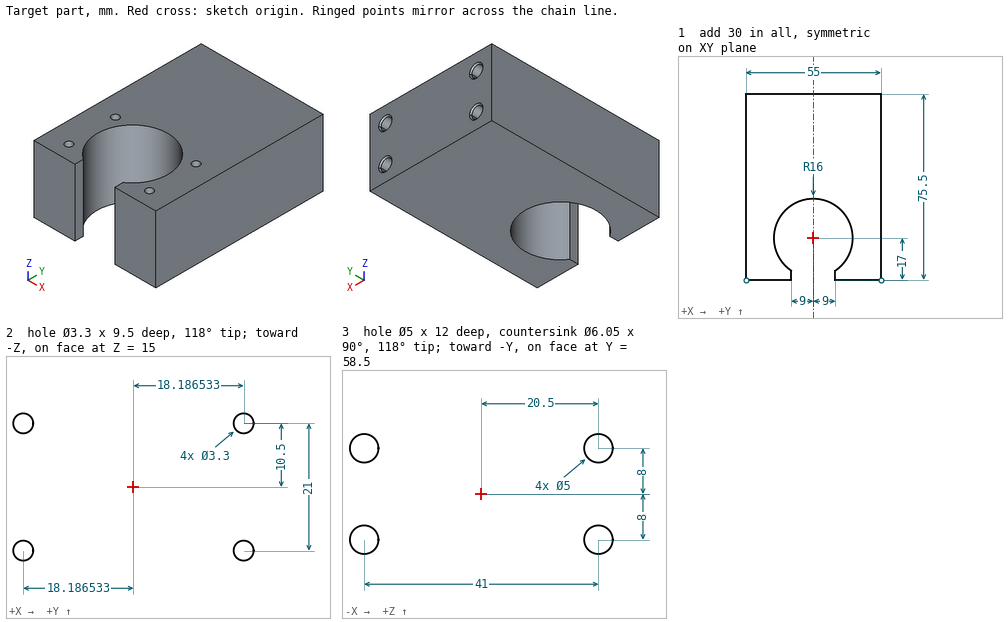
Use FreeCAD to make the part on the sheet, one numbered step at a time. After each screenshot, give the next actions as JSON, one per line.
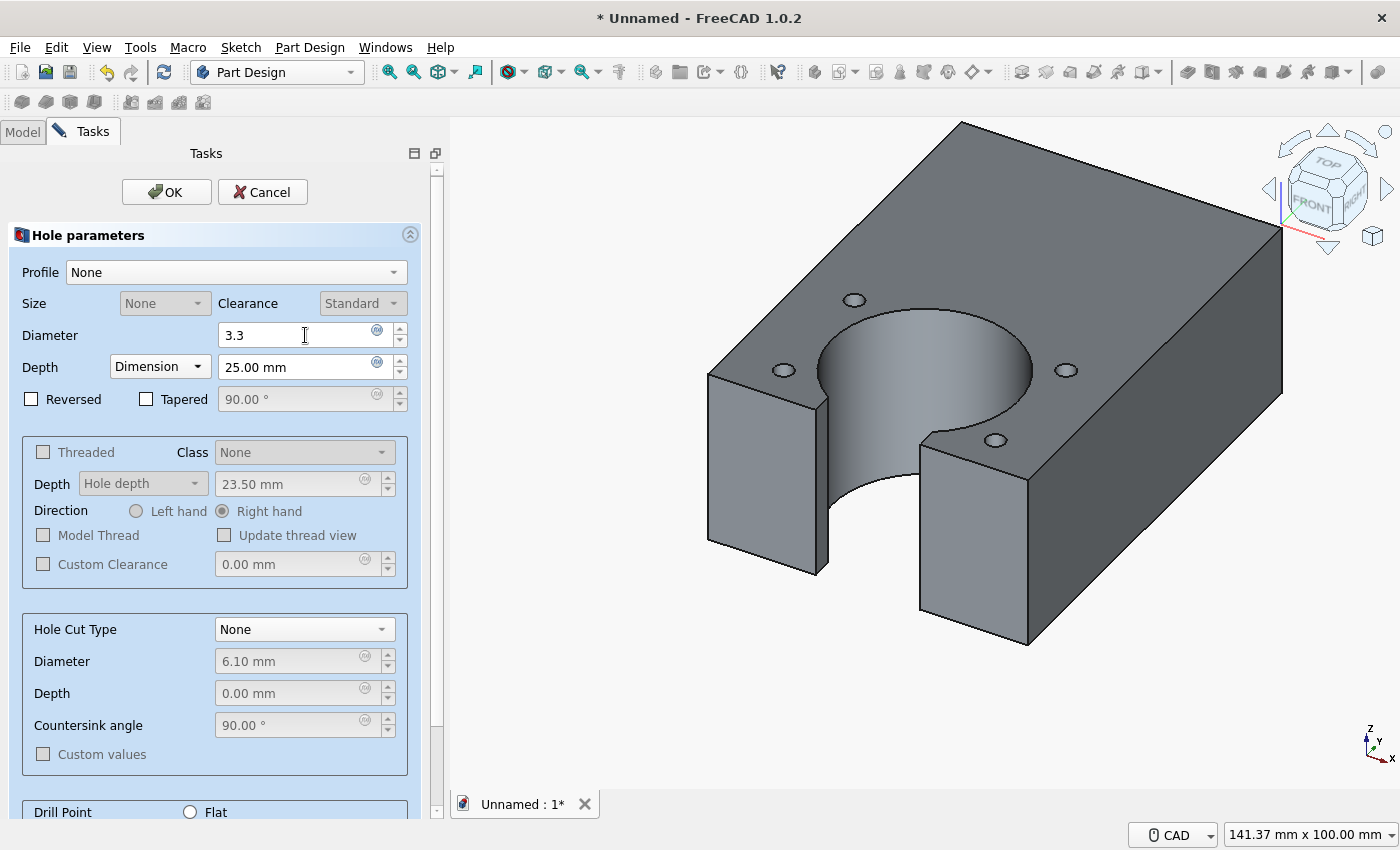
{"action": "triple_click", "coordinate": [305, 367]}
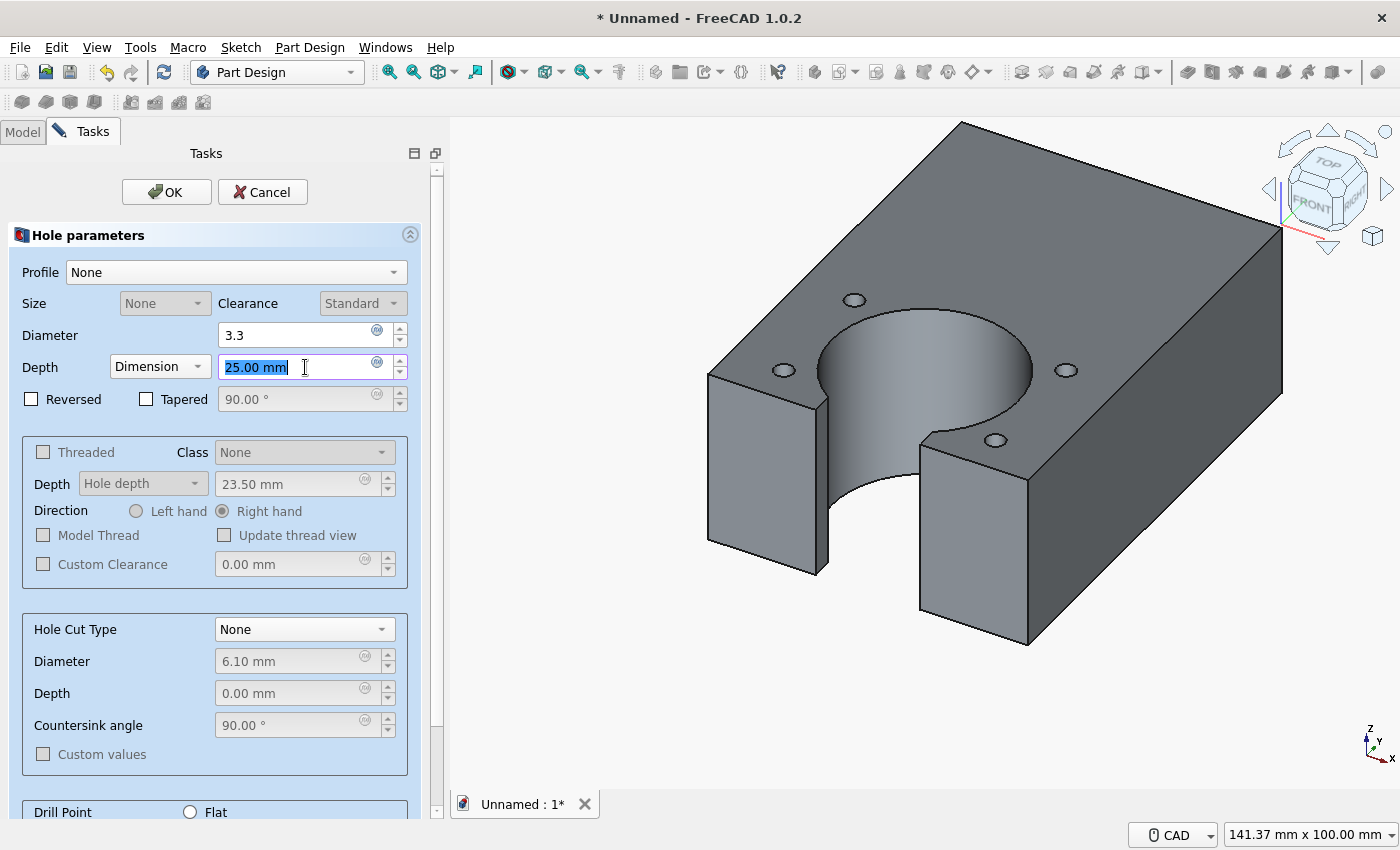
{"action": "type", "text": "9.5"}
{"action": "key", "text": "Tab"}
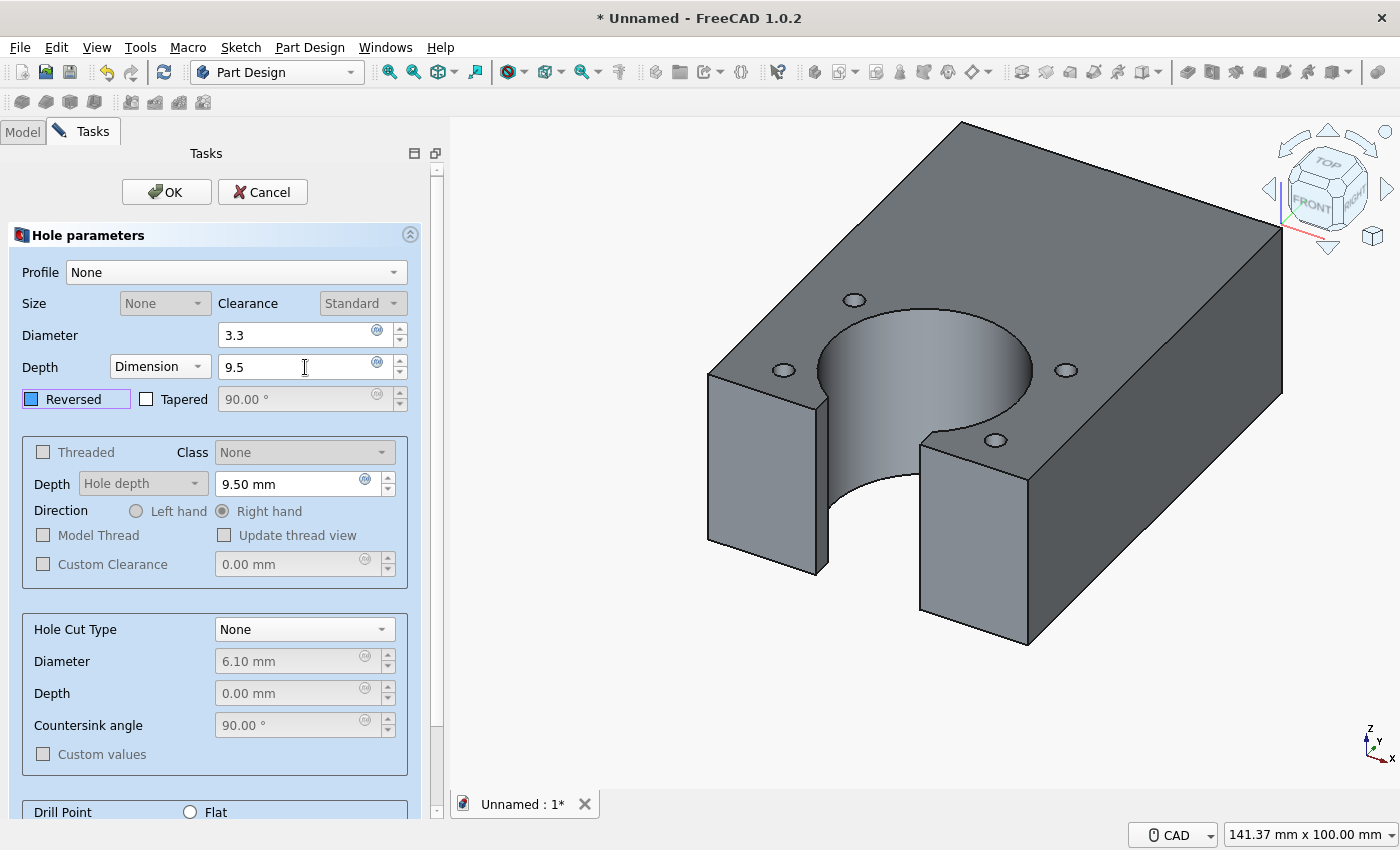
{"action": "left_click", "coordinate": [167, 192]}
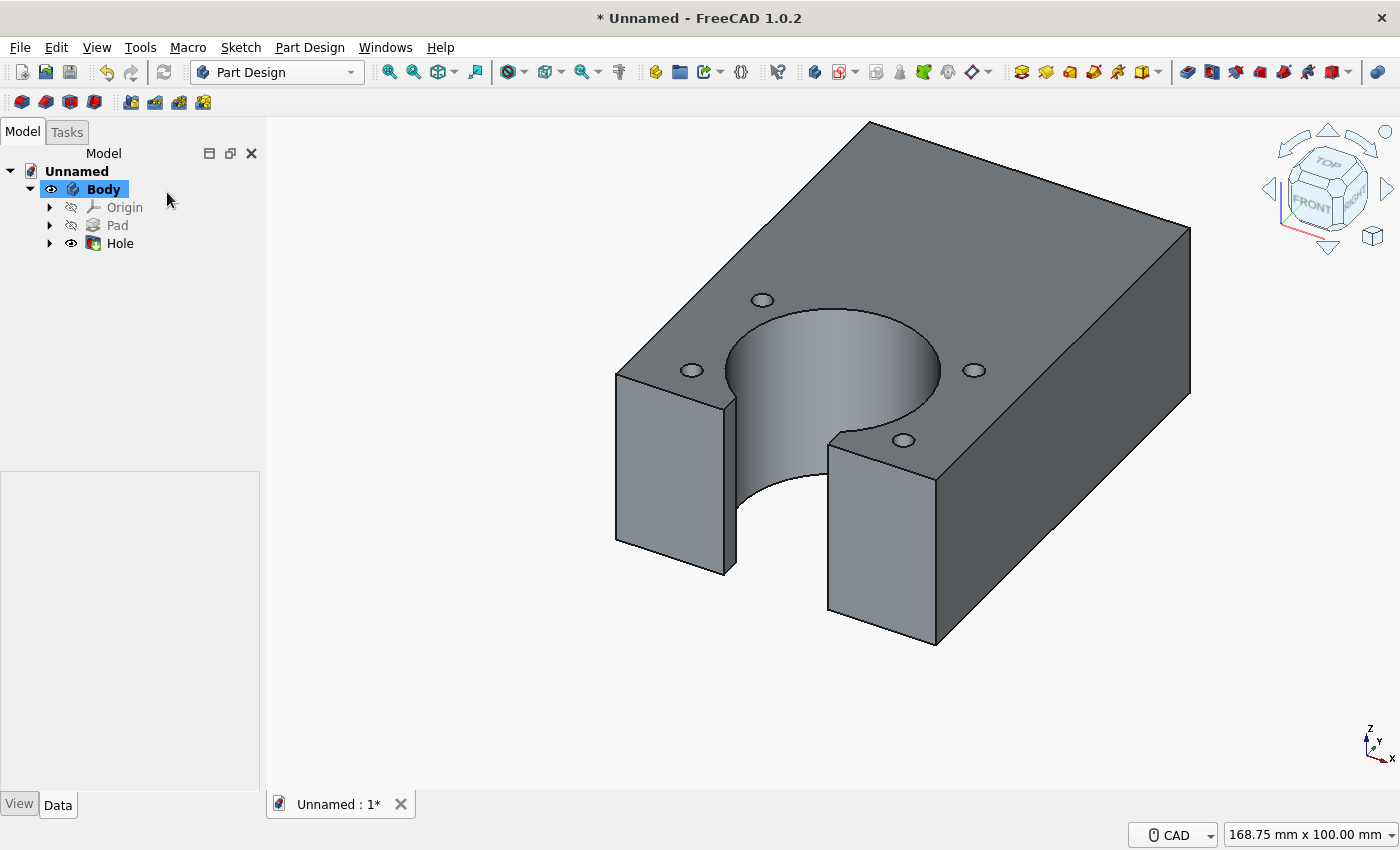
{"action": "key", "text": "4"}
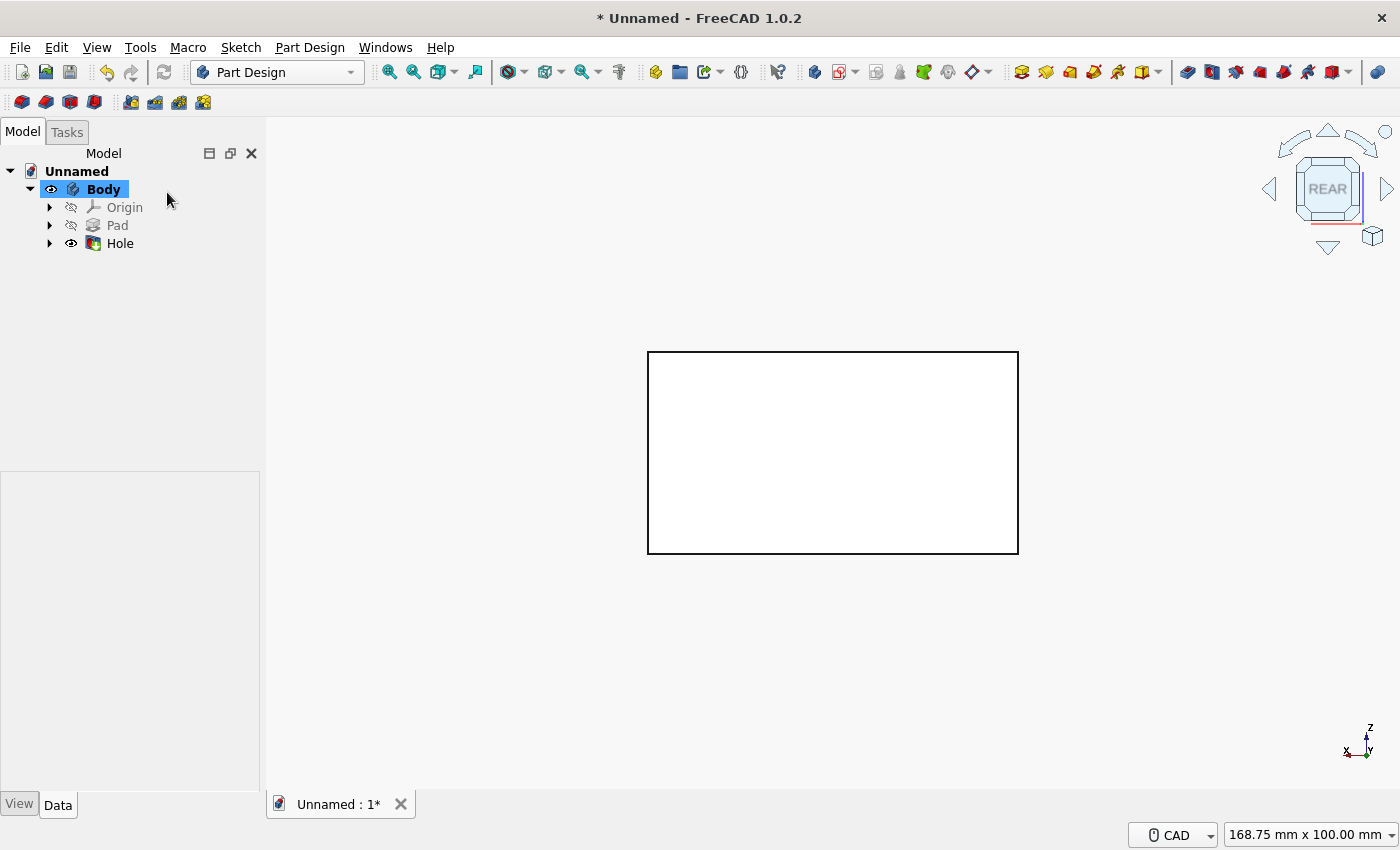
{"action": "left_click", "coordinate": [390, 72]}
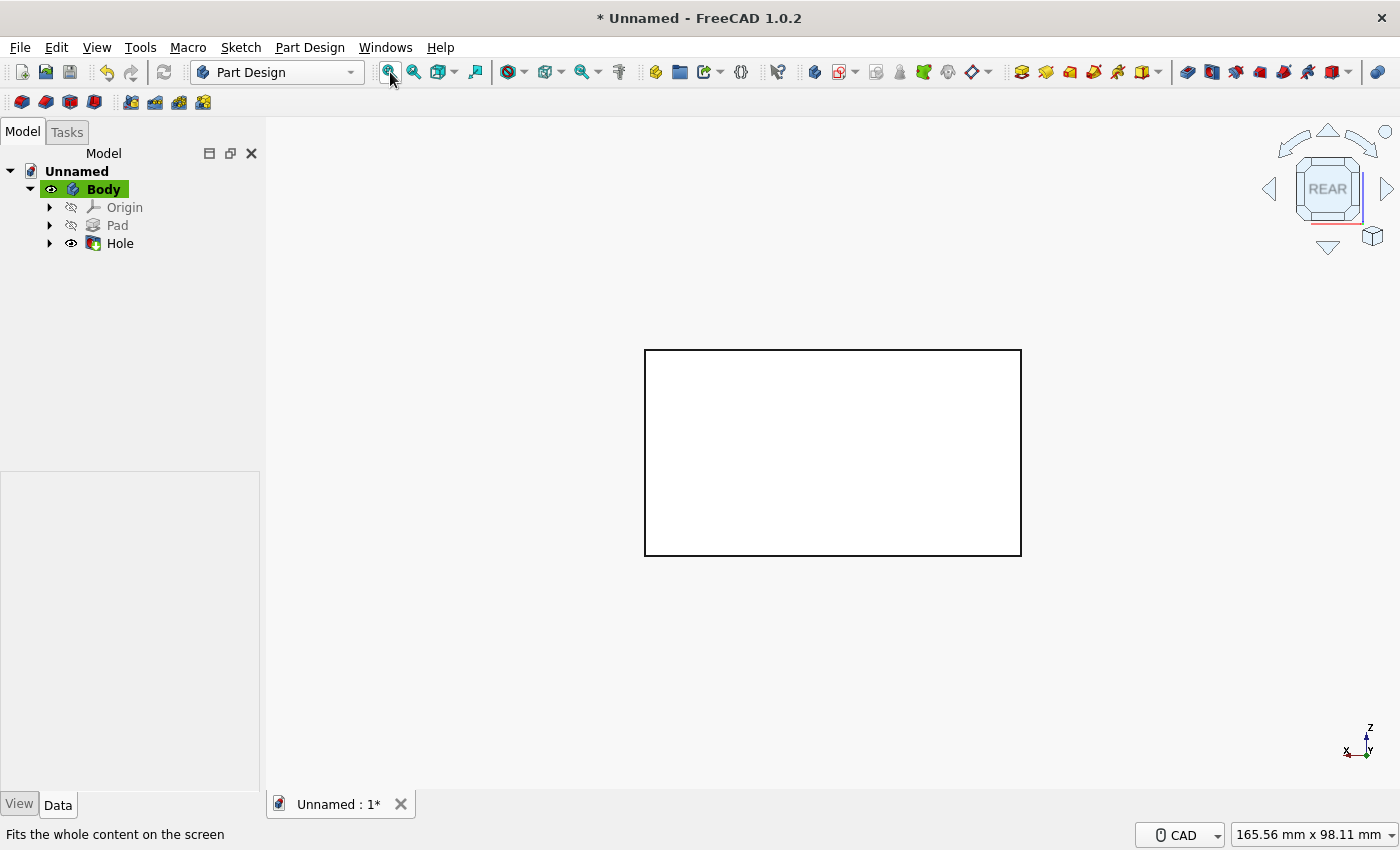
{"action": "left_click", "coordinate": [779, 452]}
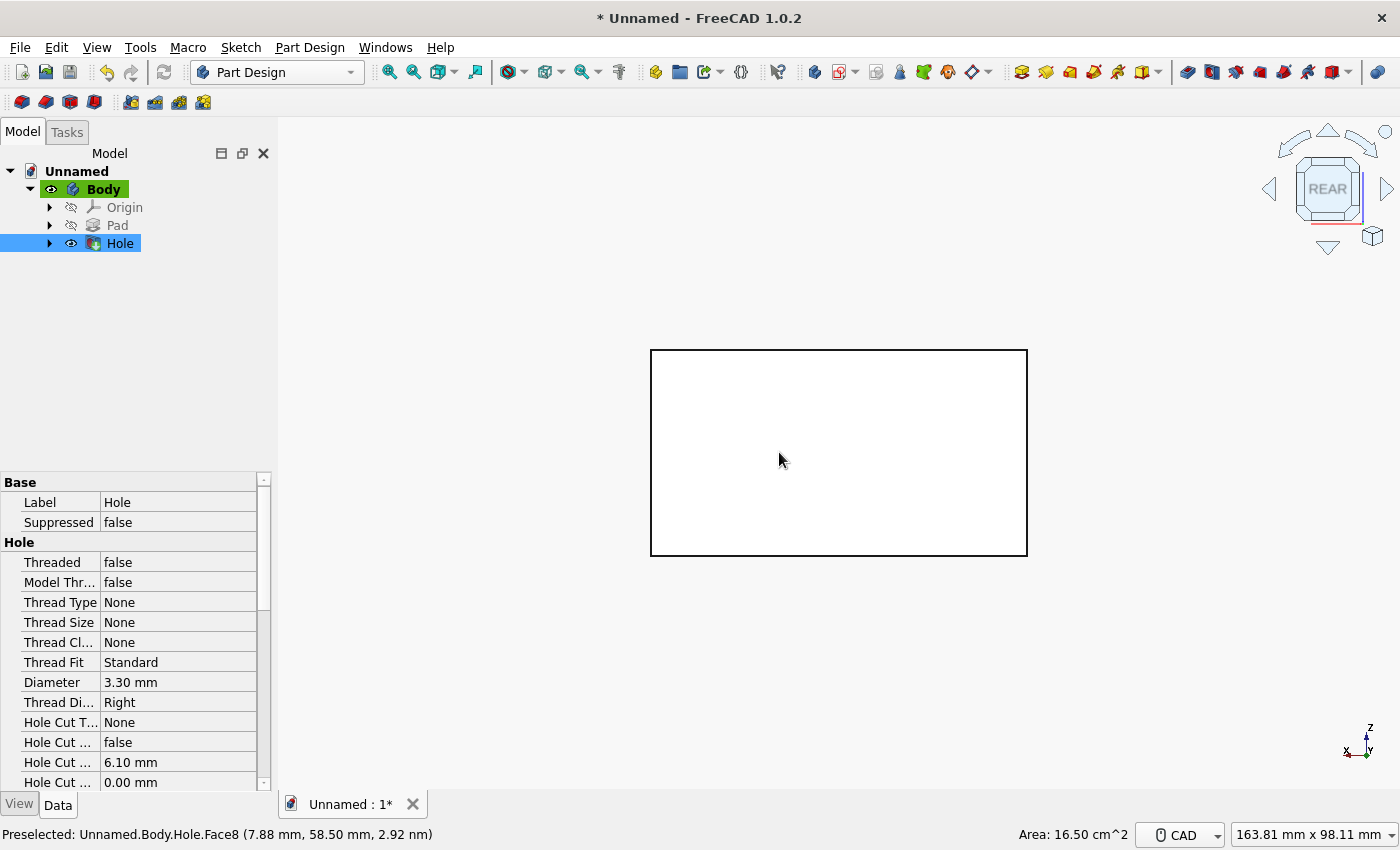
{"action": "left_click", "coordinate": [840, 72]}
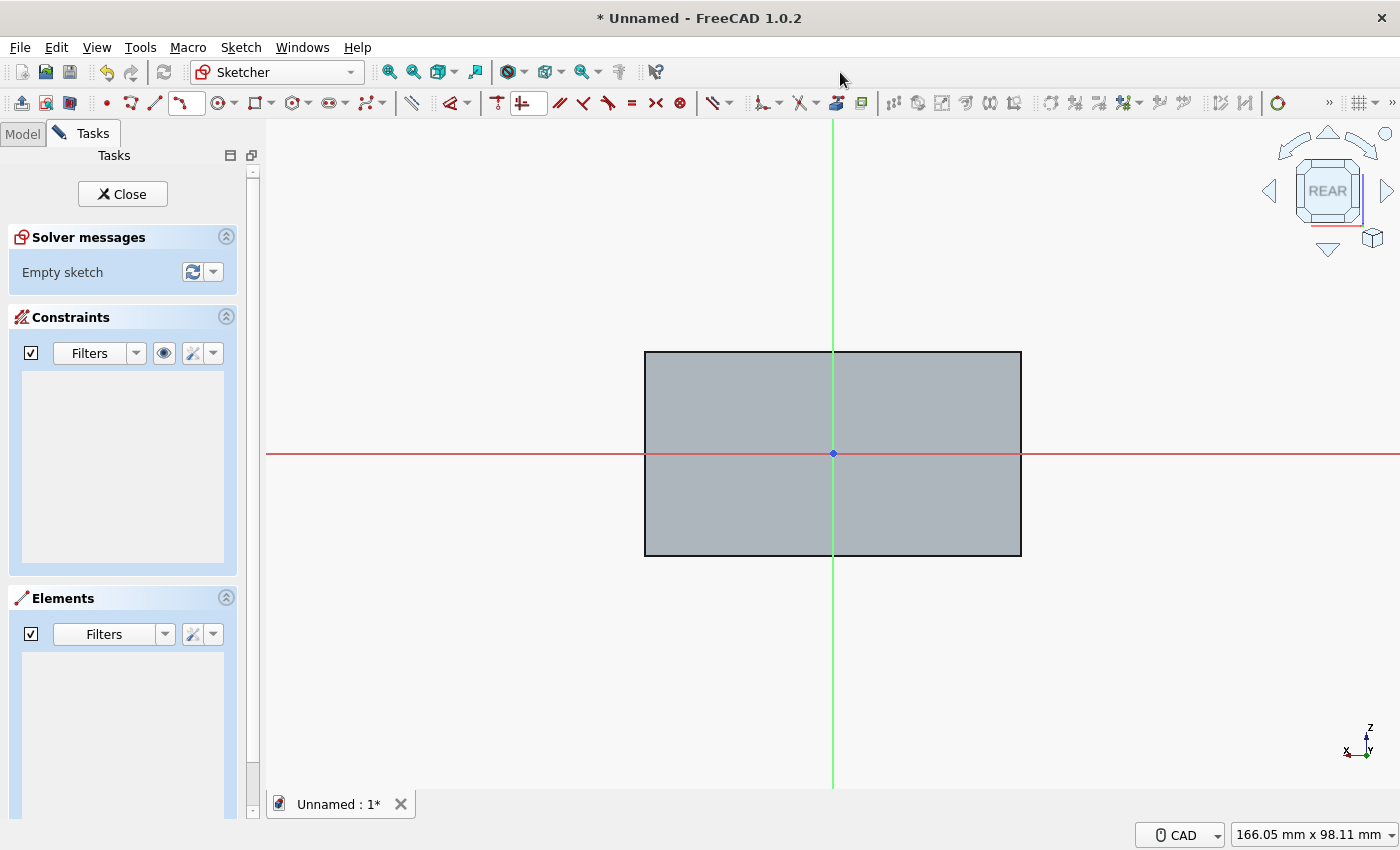
{"action": "scroll", "coordinate": [889, 454], "scroll_direction": "up", "scroll_amount": 4}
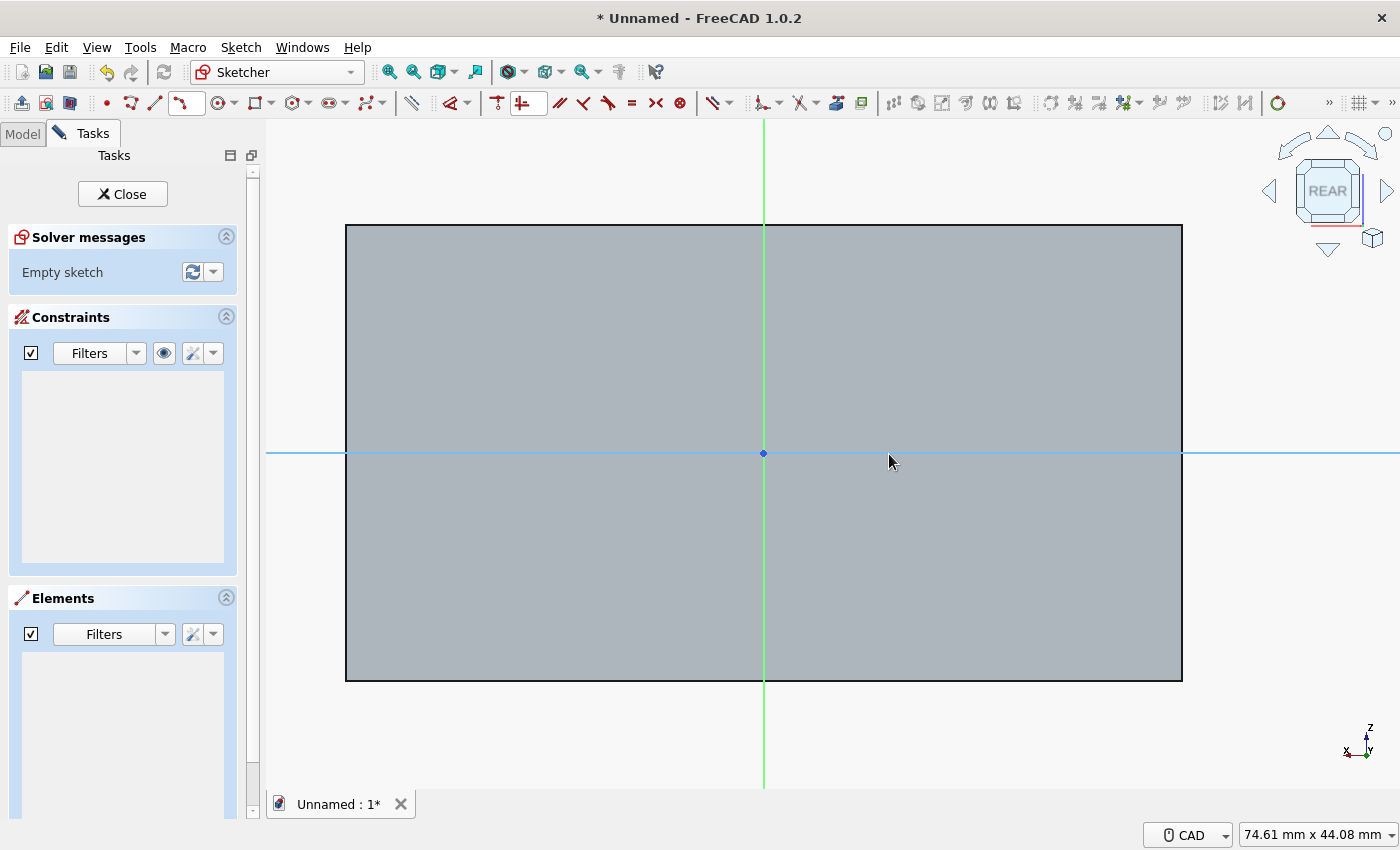
{"action": "left_click", "coordinate": [218, 104]}